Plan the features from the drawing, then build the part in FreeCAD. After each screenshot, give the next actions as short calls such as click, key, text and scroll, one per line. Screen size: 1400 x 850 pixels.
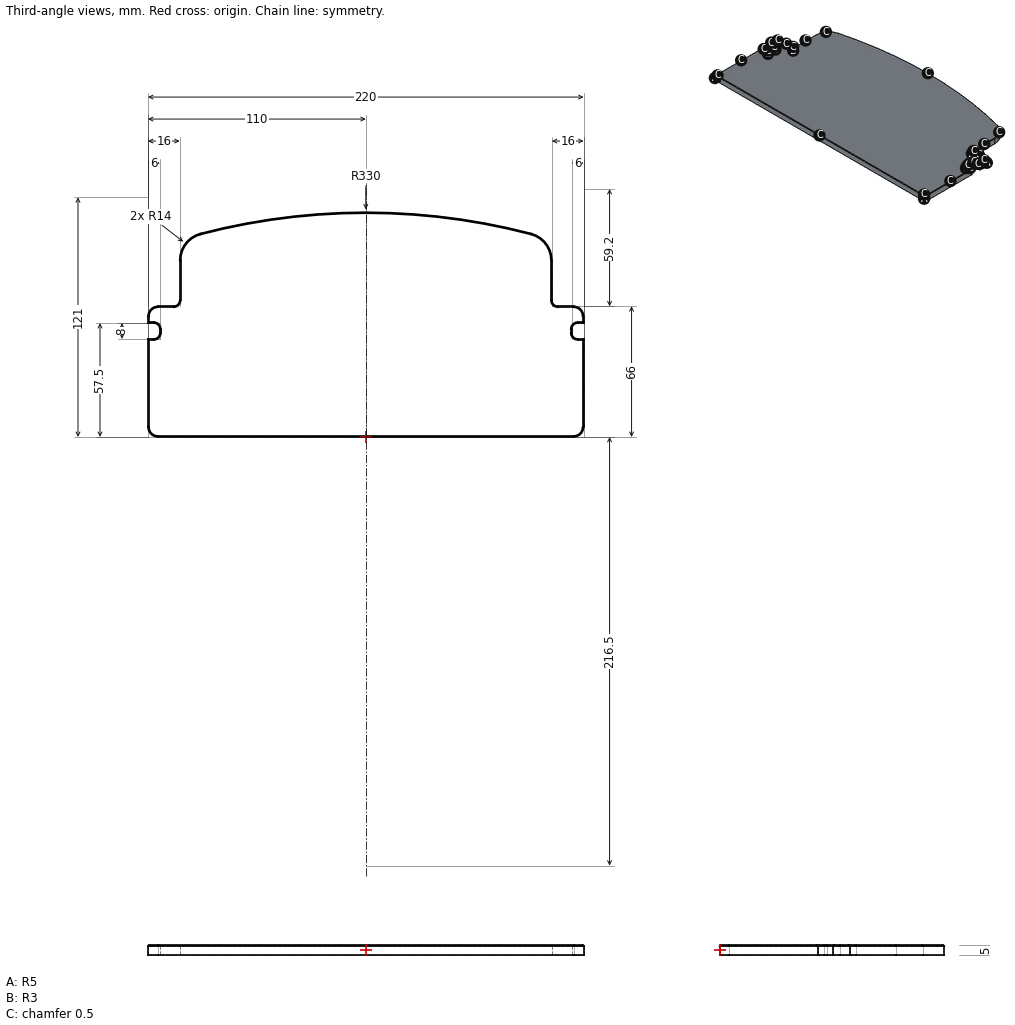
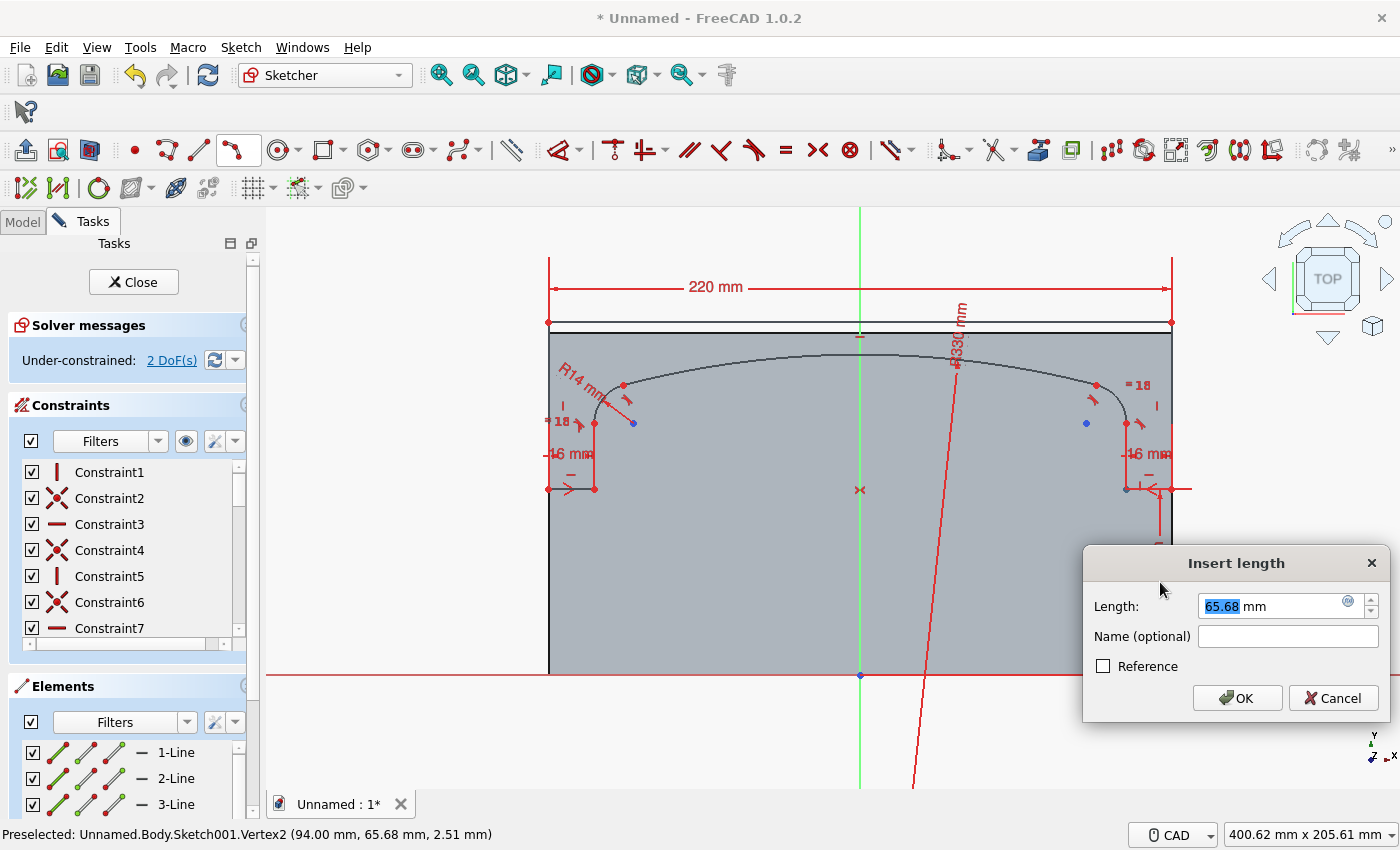
text(66)
key(Return)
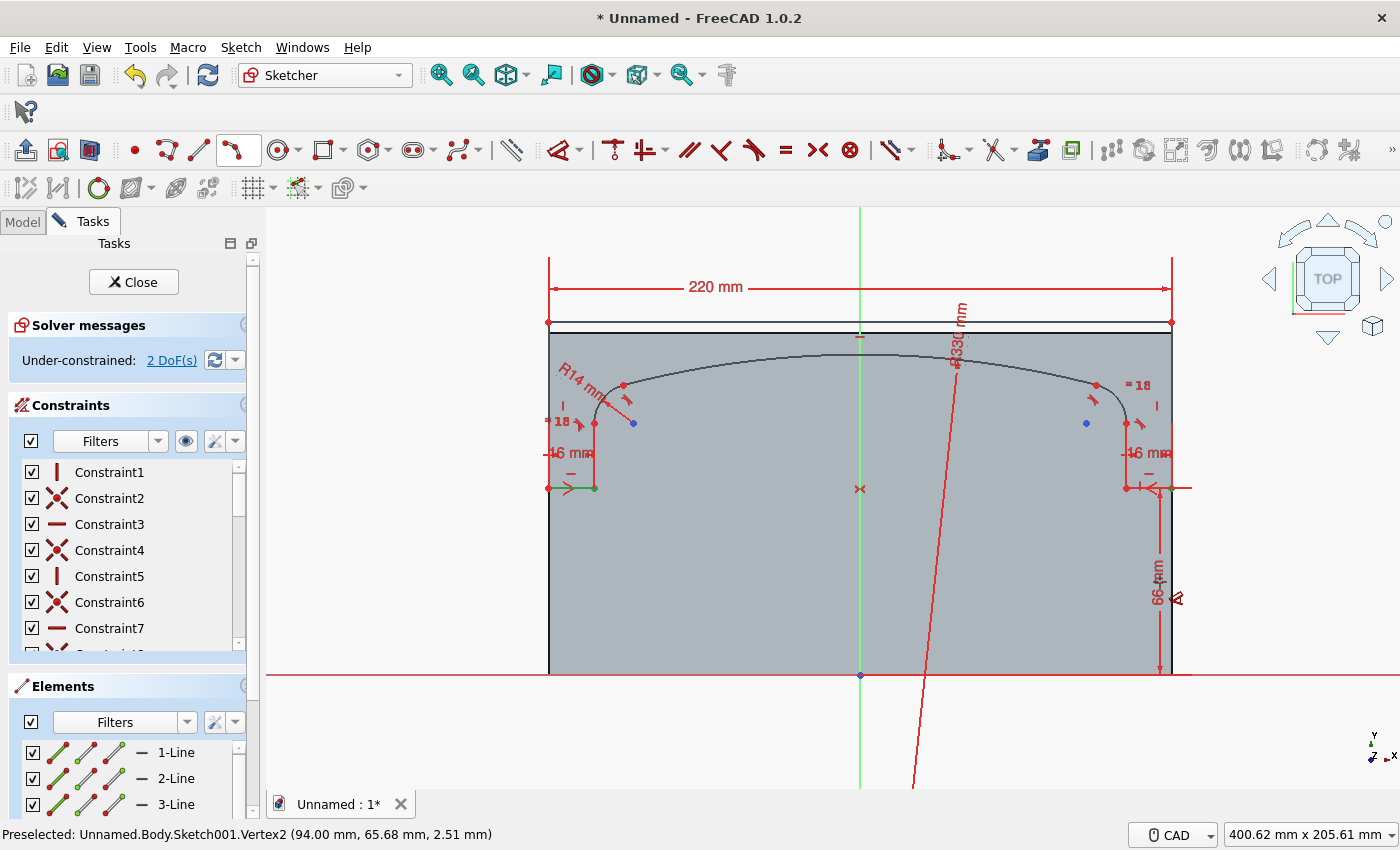
click(1172, 439)
click(1206, 405)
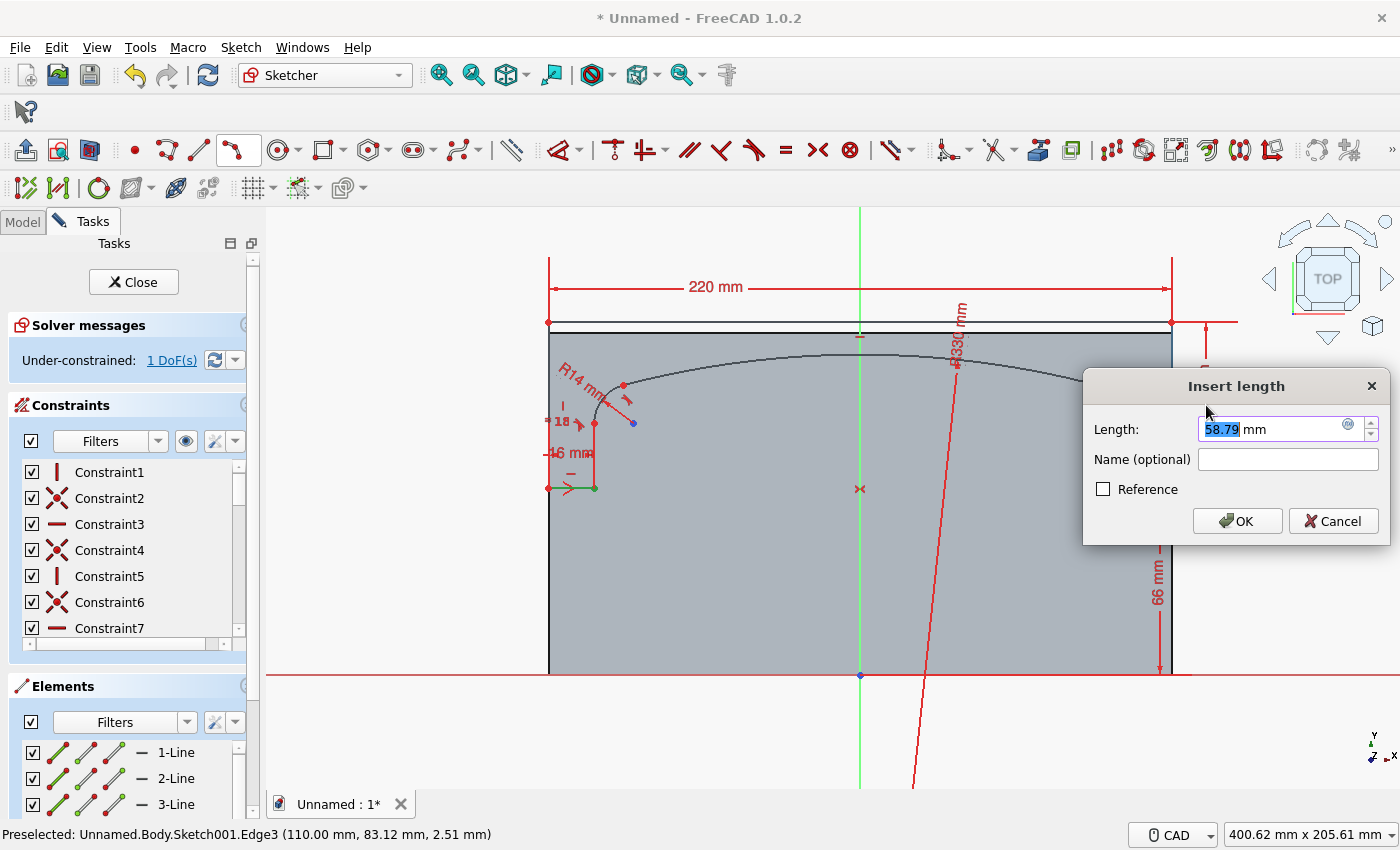
text(59.2)
key(Return)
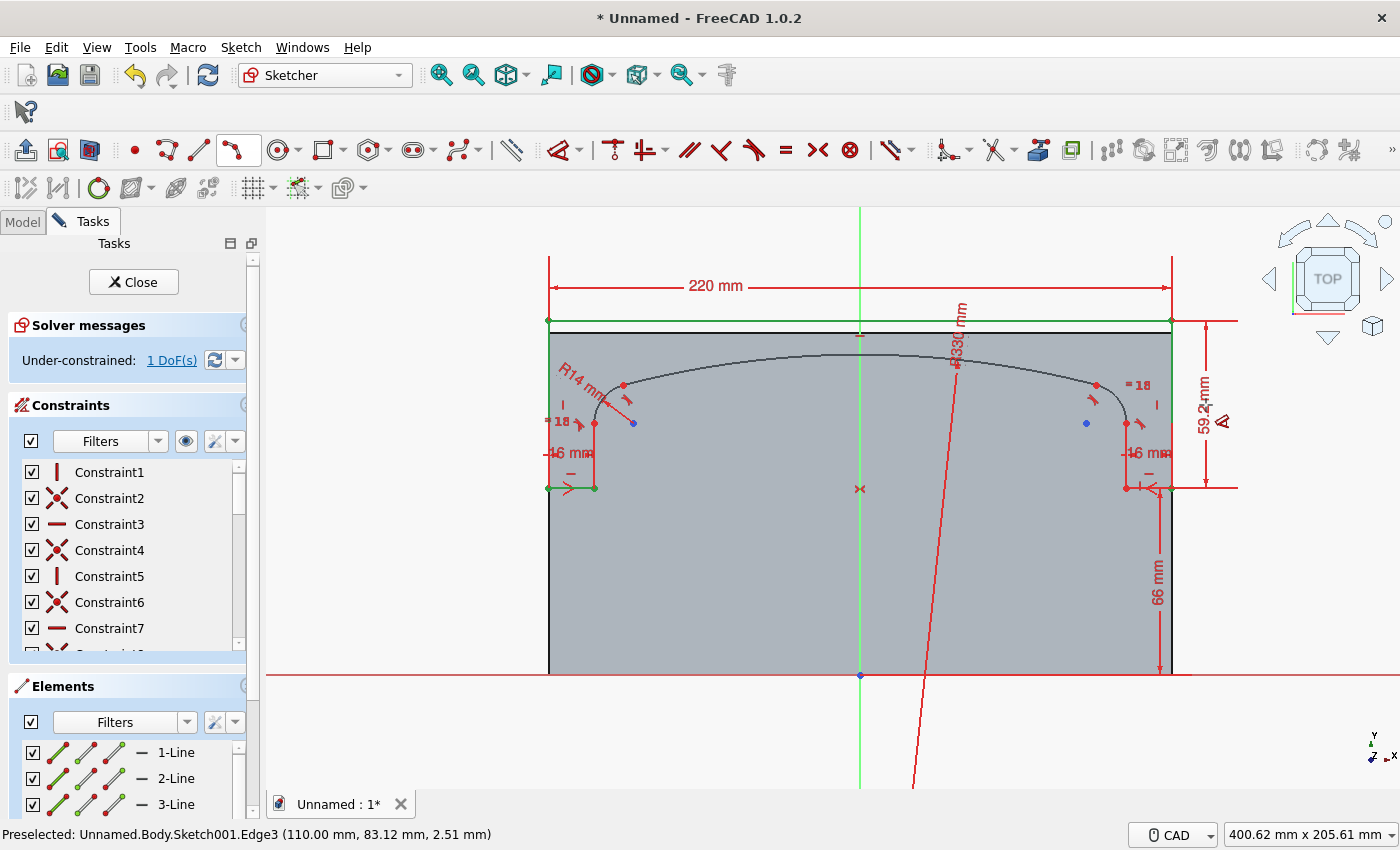
scroll(709, 319, down, 5)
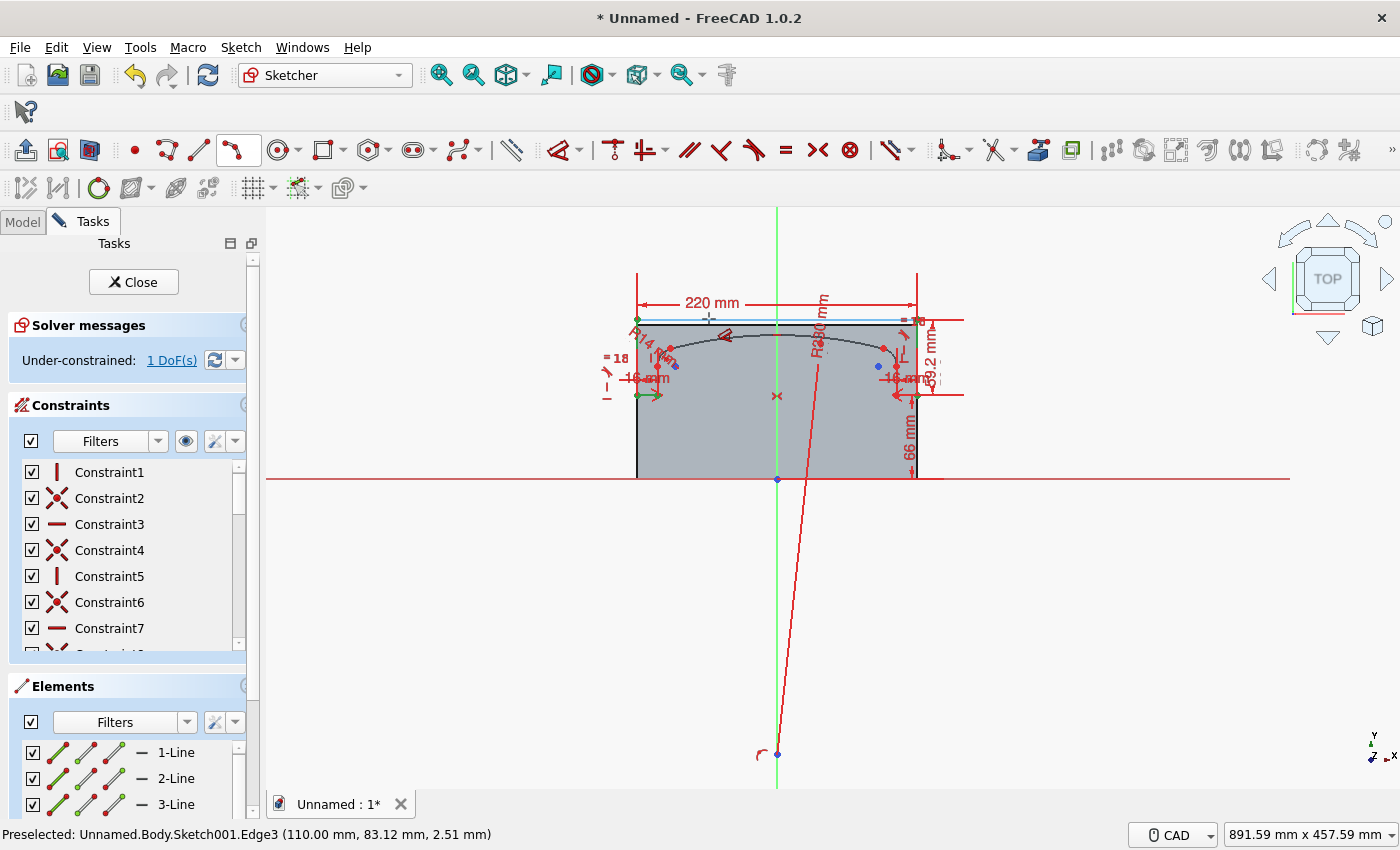
click(765, 676)
click(799, 563)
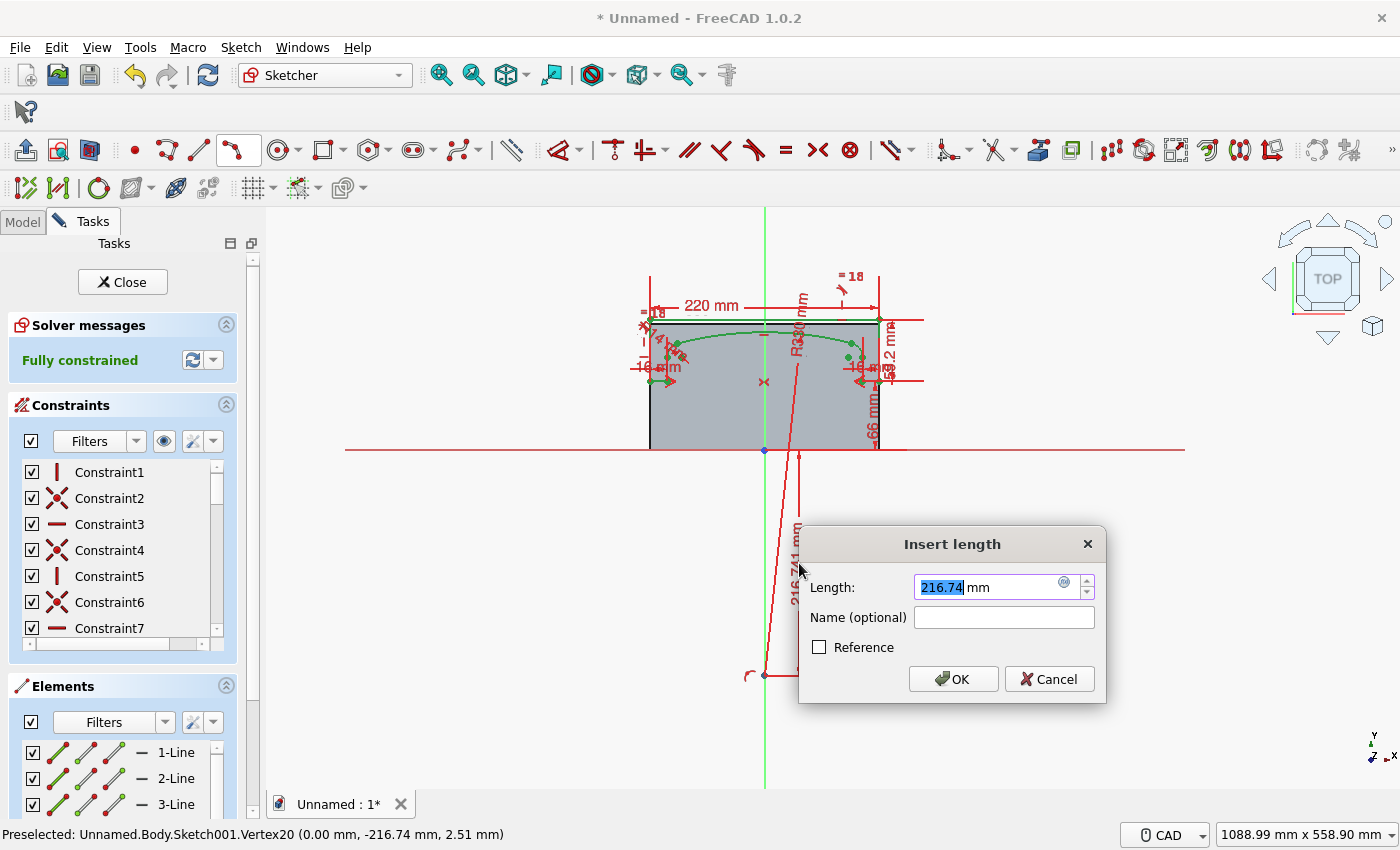
text(216.5)
key(Return)
key(Escape)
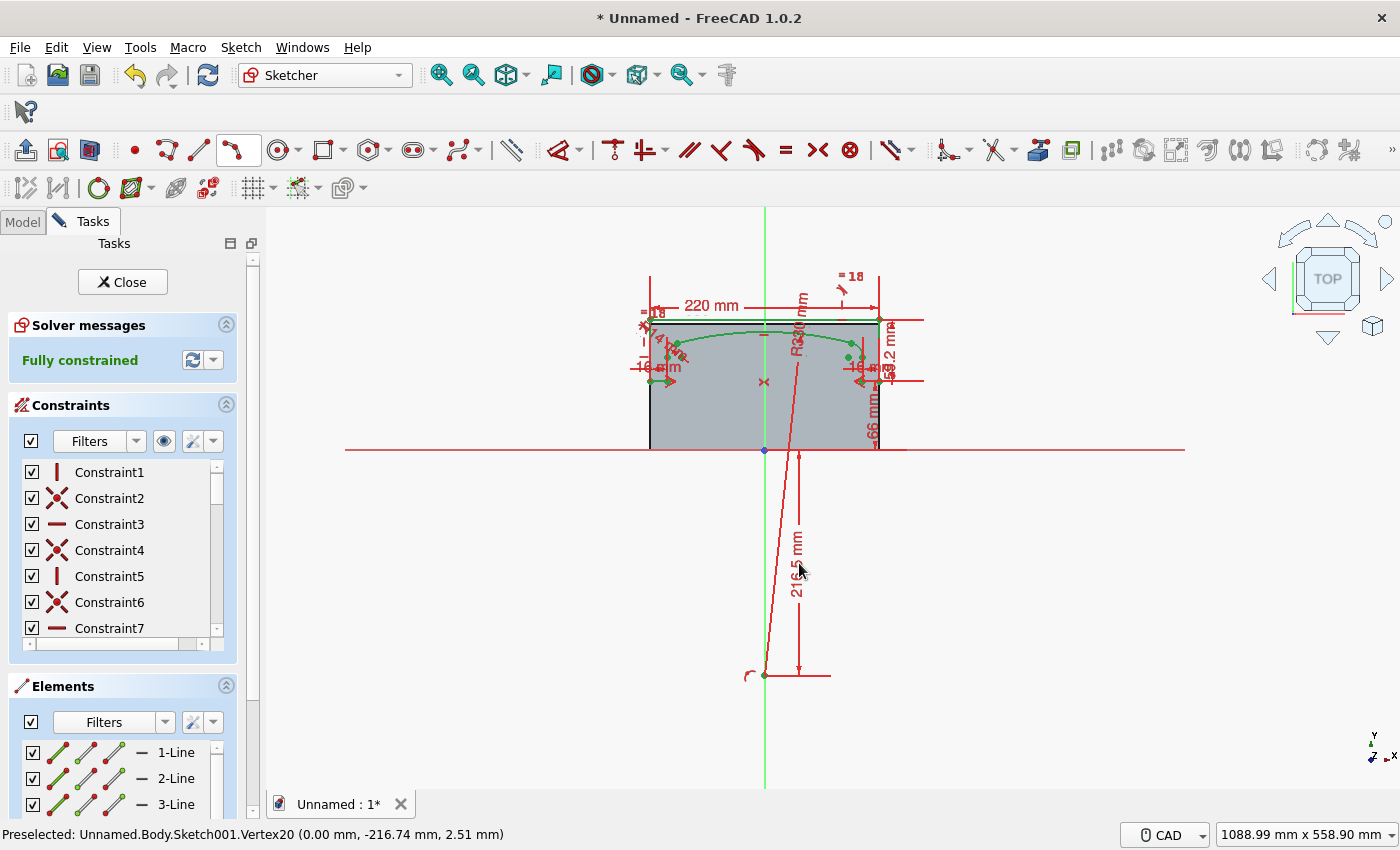
click(123, 282)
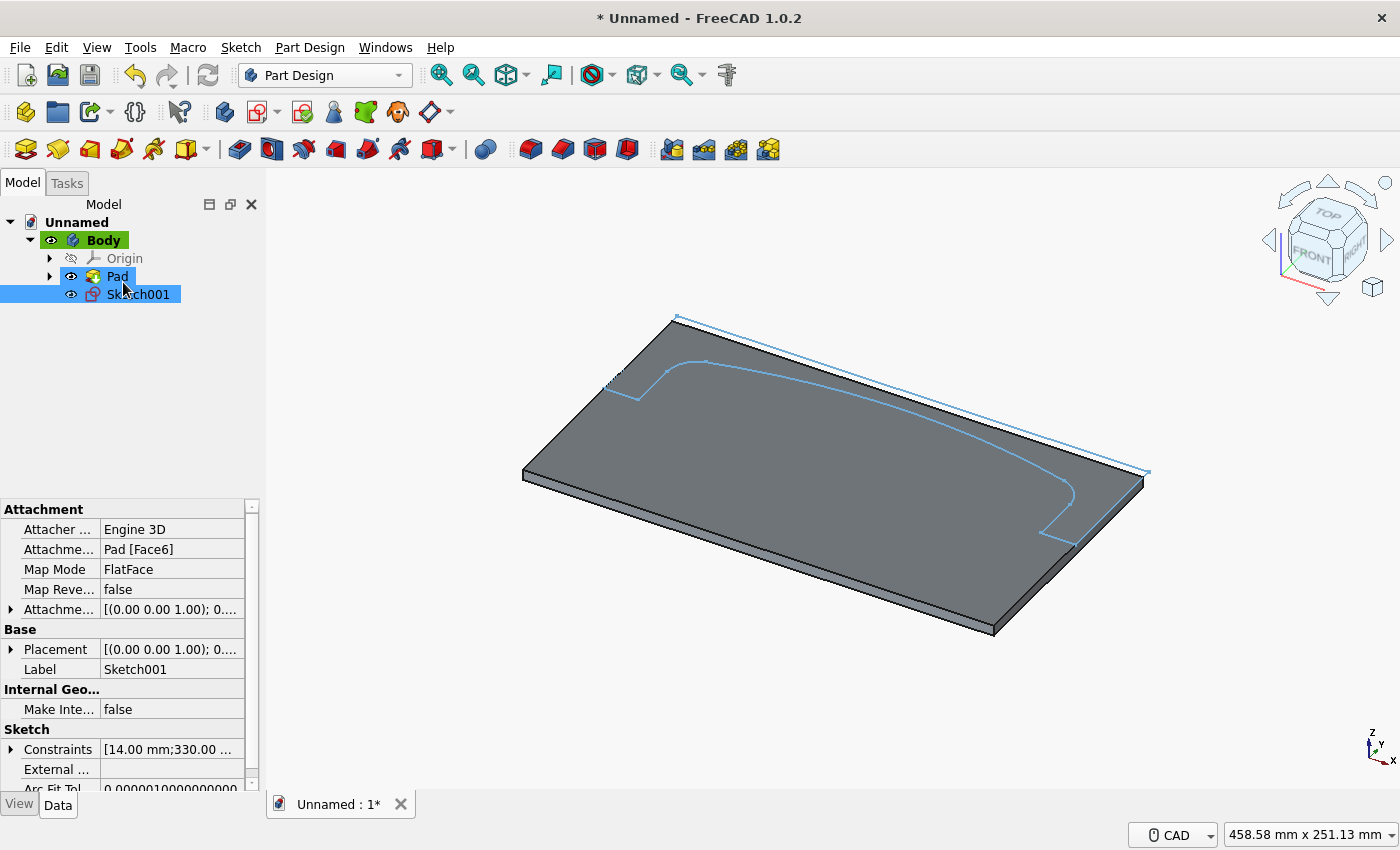
click(240, 150)